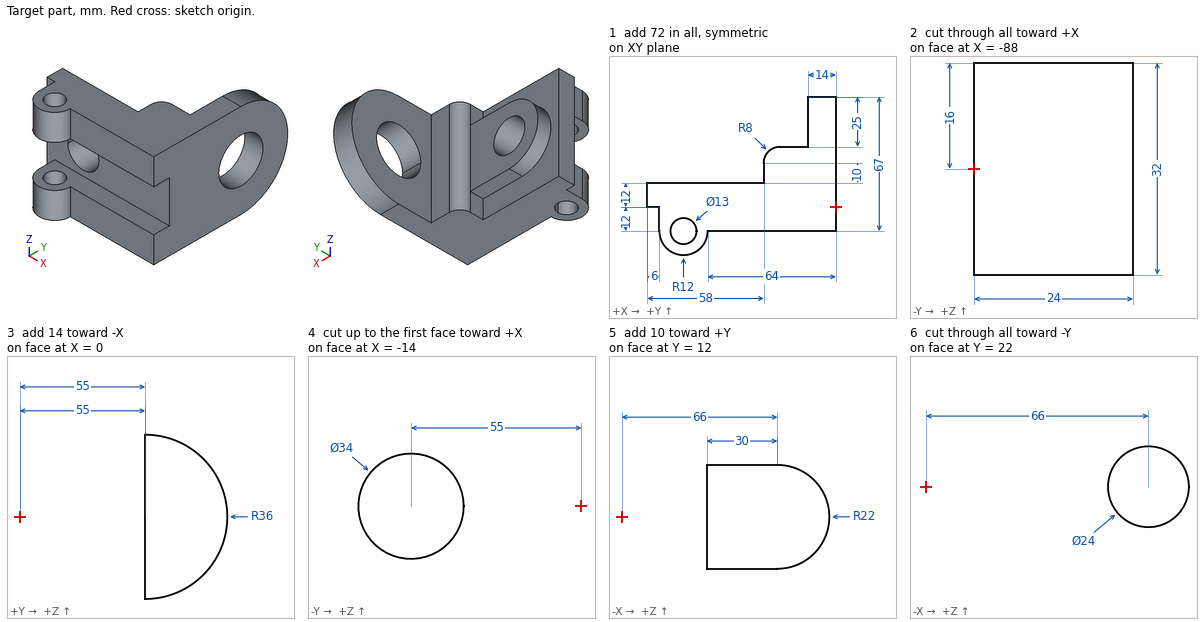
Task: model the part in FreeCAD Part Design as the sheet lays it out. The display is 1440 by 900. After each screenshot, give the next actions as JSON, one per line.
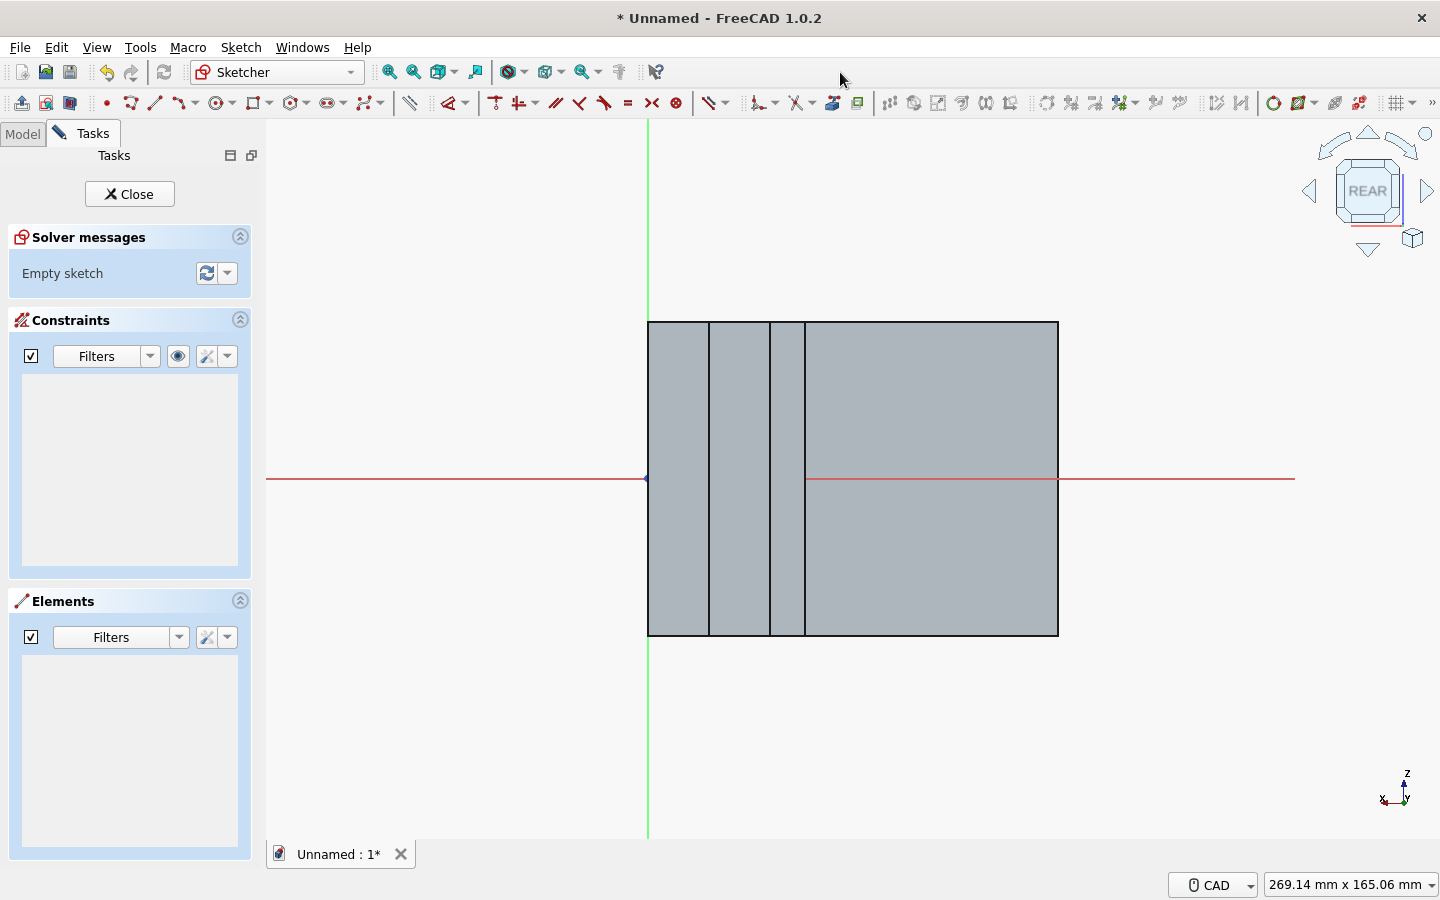
{"action": "scroll", "coordinate": [907, 479], "scroll_direction": "up", "scroll_amount": 3}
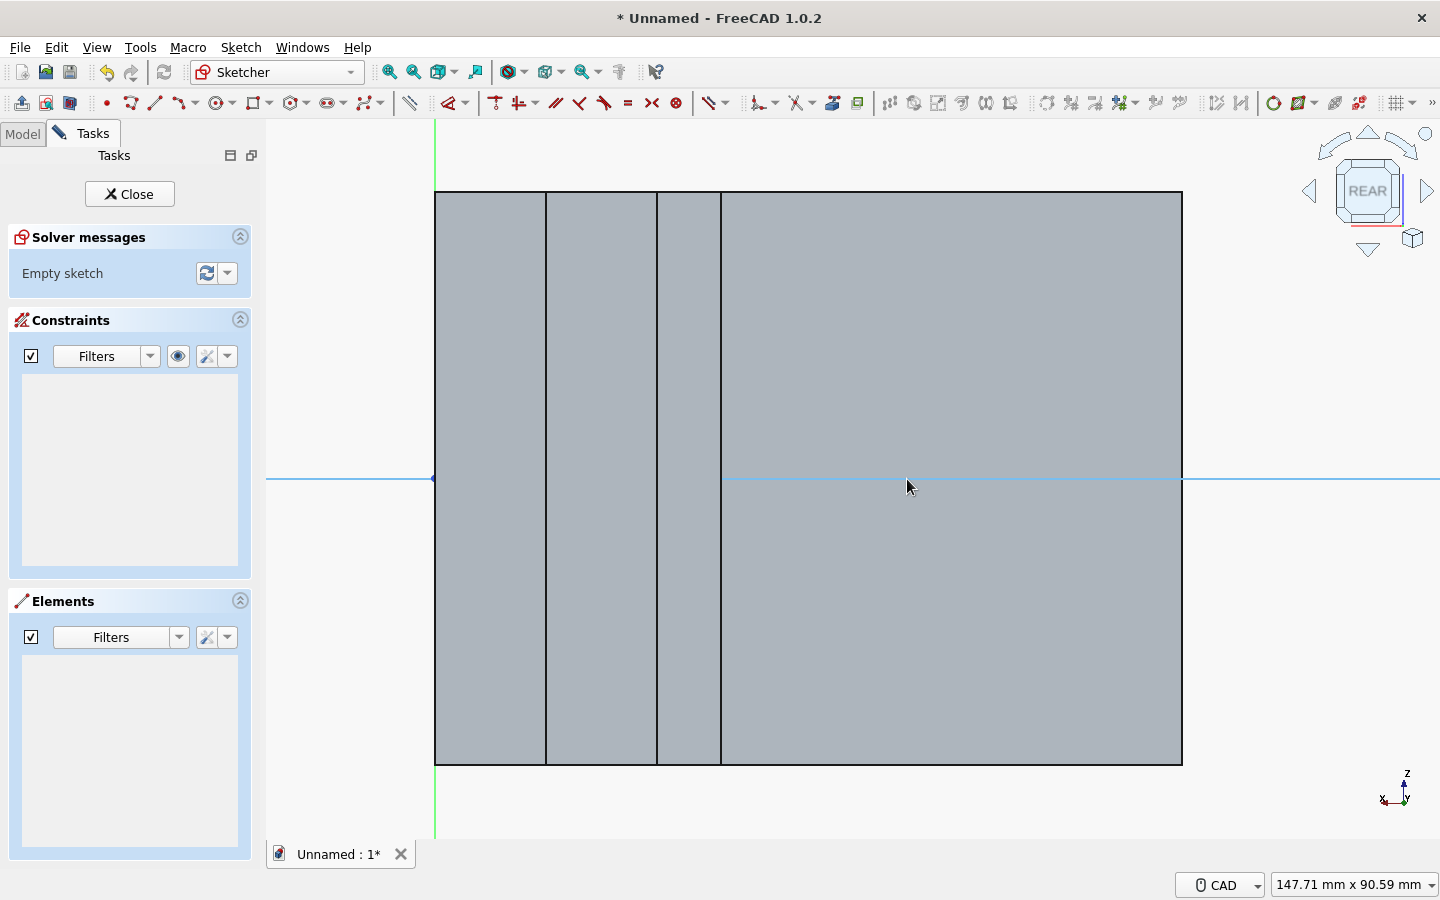
{"action": "left_click", "coordinate": [132, 104]}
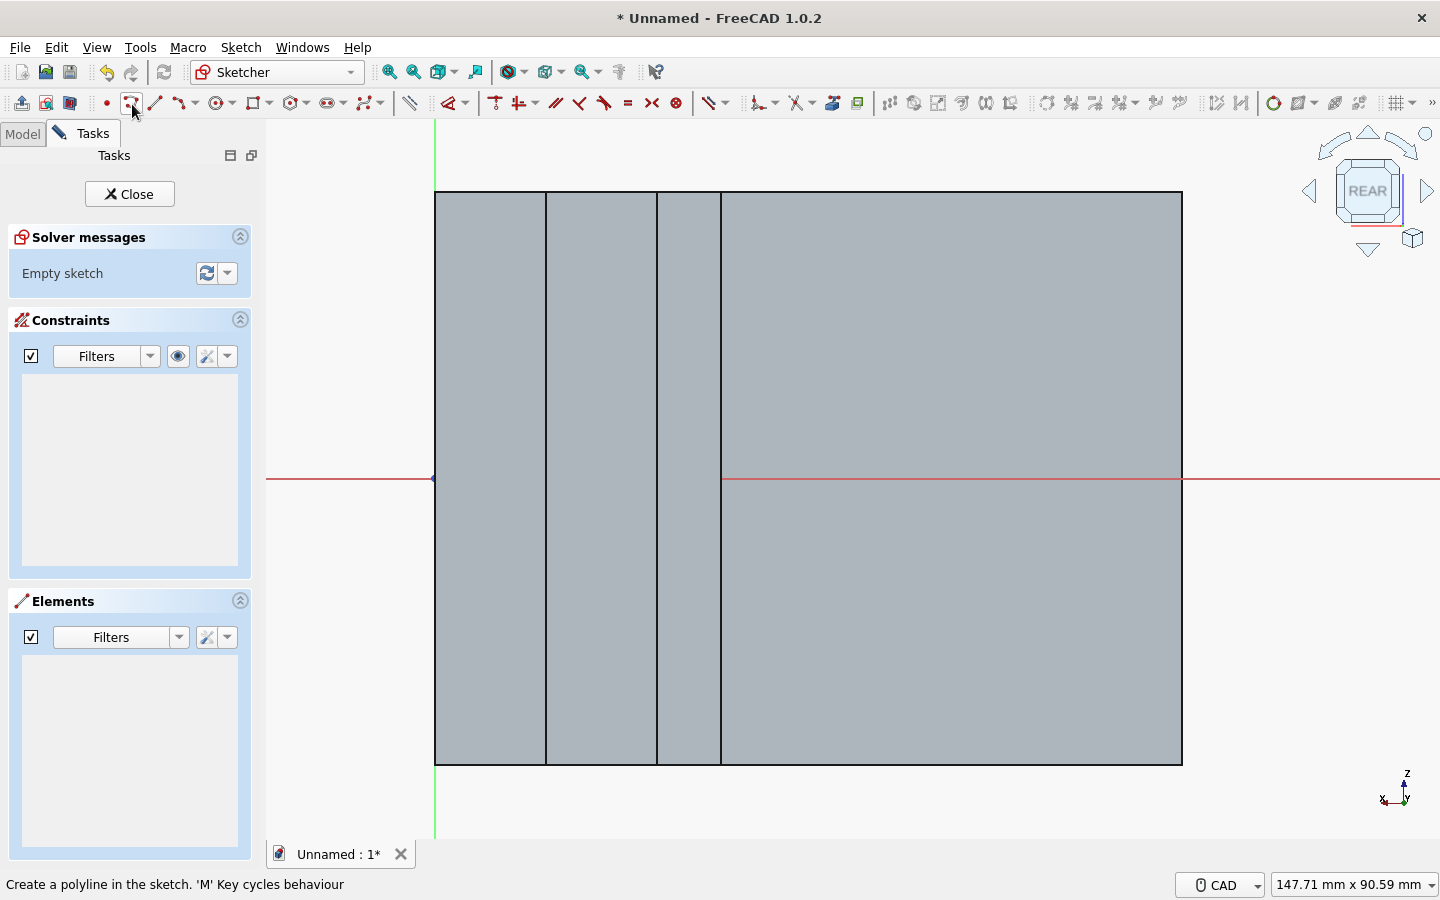
{"action": "left_click", "coordinate": [959, 304]}
{"action": "left_click", "coordinate": [721, 304]}
{"action": "left_click", "coordinate": [721, 653]}
{"action": "left_click", "coordinate": [959, 653]}
{"action": "right_click", "coordinate": [959, 653]}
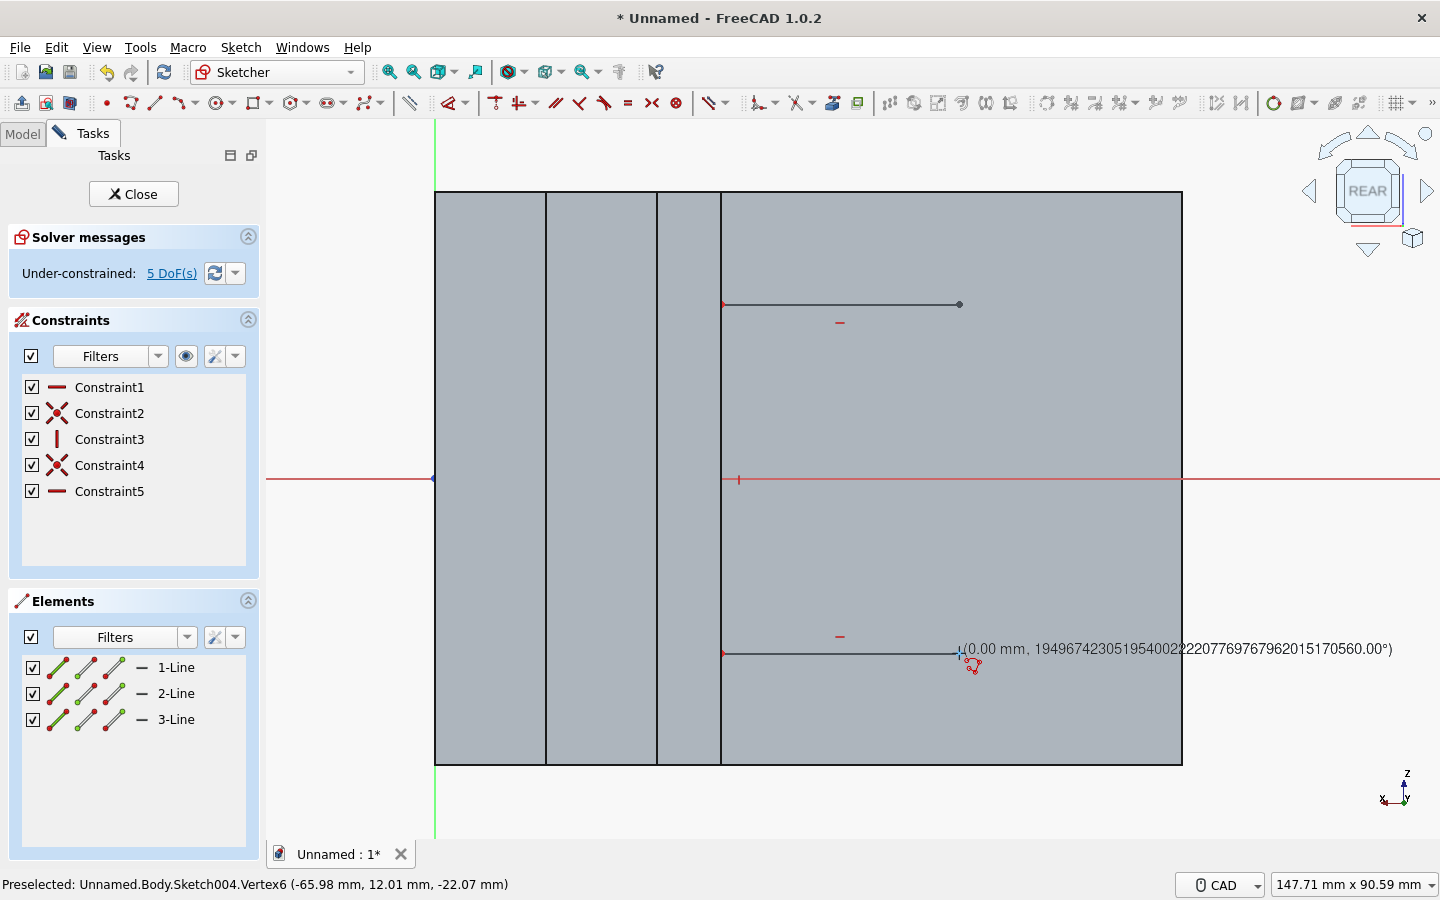
{"action": "left_click", "coordinate": [180, 104]}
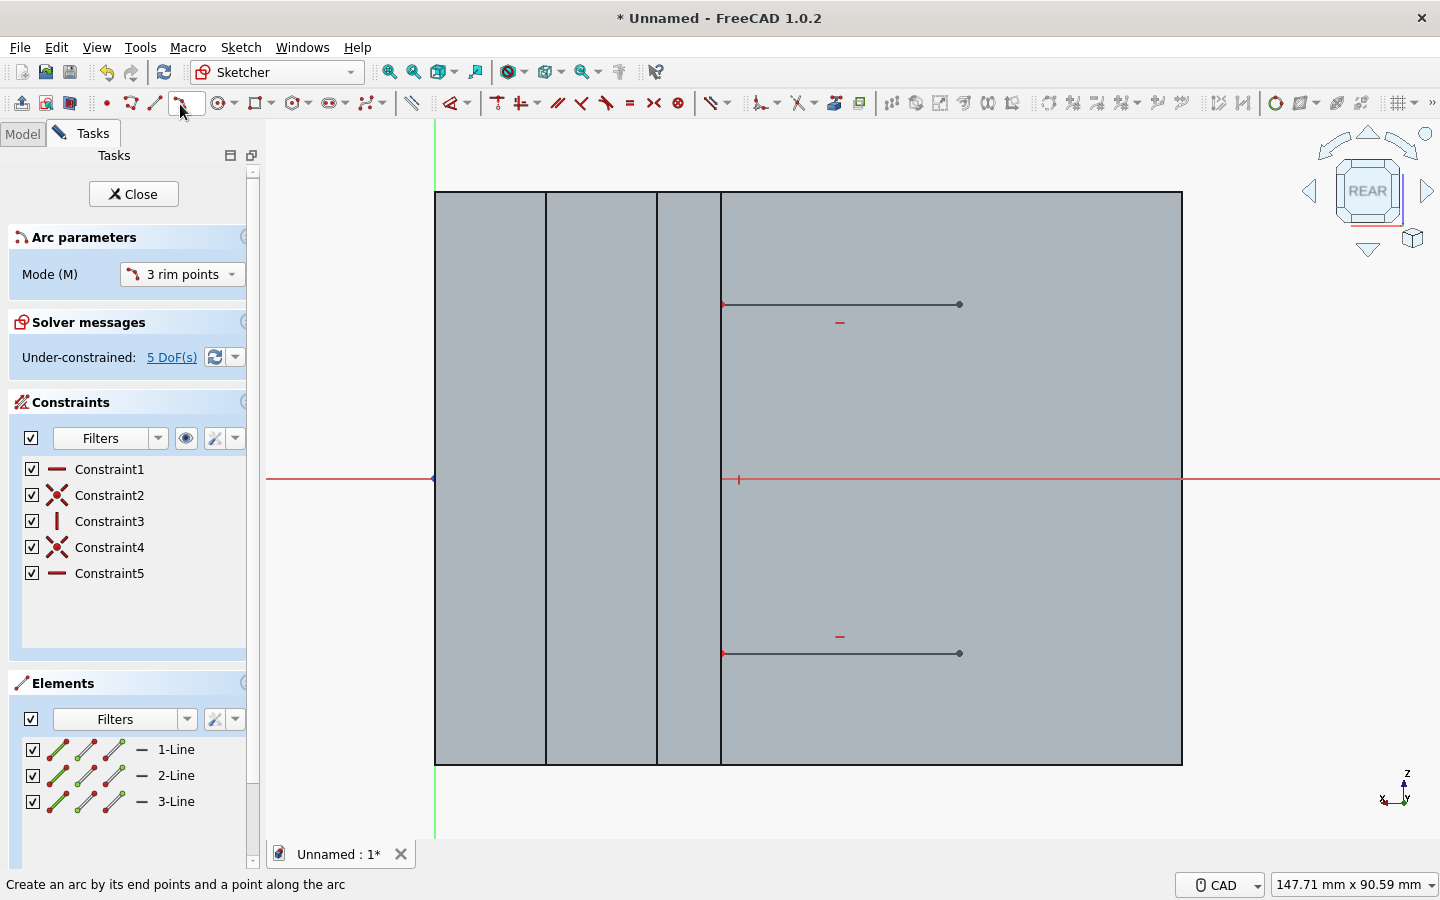
{"action": "left_click", "coordinate": [959, 654]}
{"action": "left_click", "coordinate": [959, 305]}
{"action": "left_click", "coordinate": [1125, 533]}
{"action": "key", "text": "Escape"}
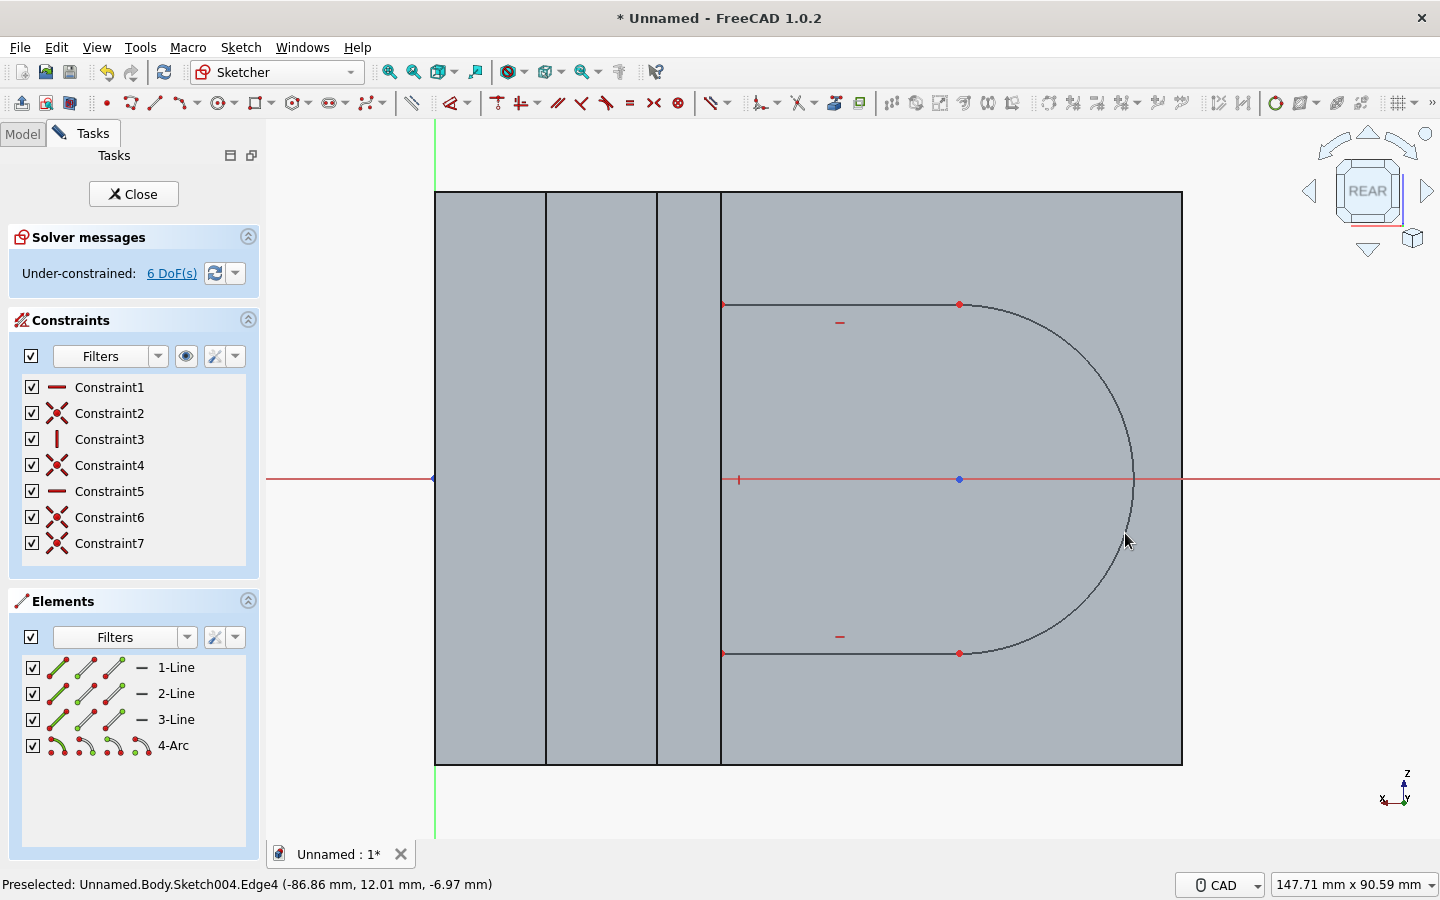
{"action": "left_click", "coordinate": [888, 305]}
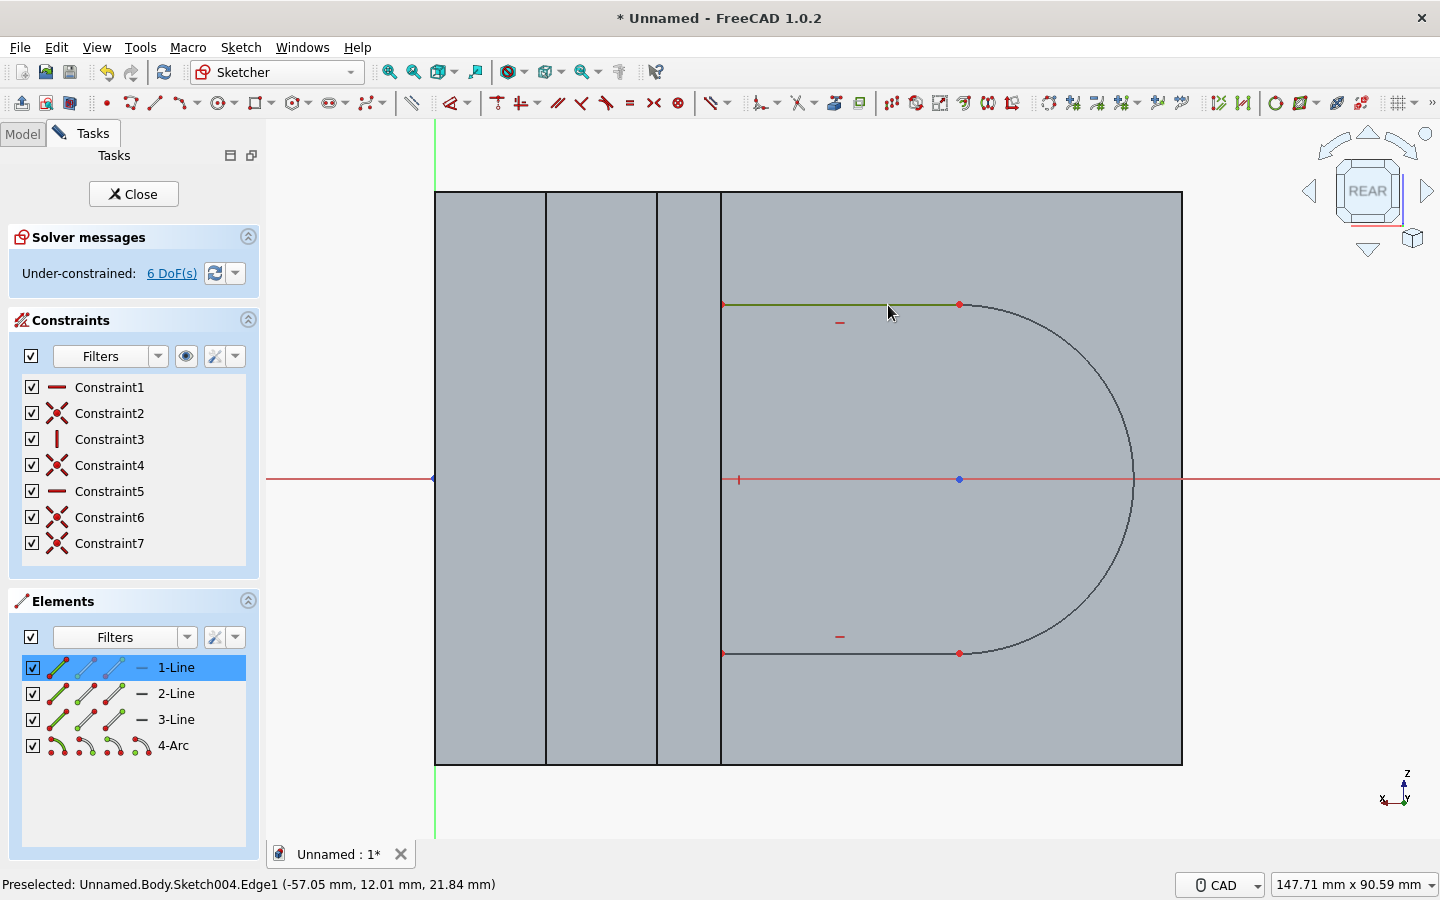
{"action": "left_click", "coordinate": [1100, 582]}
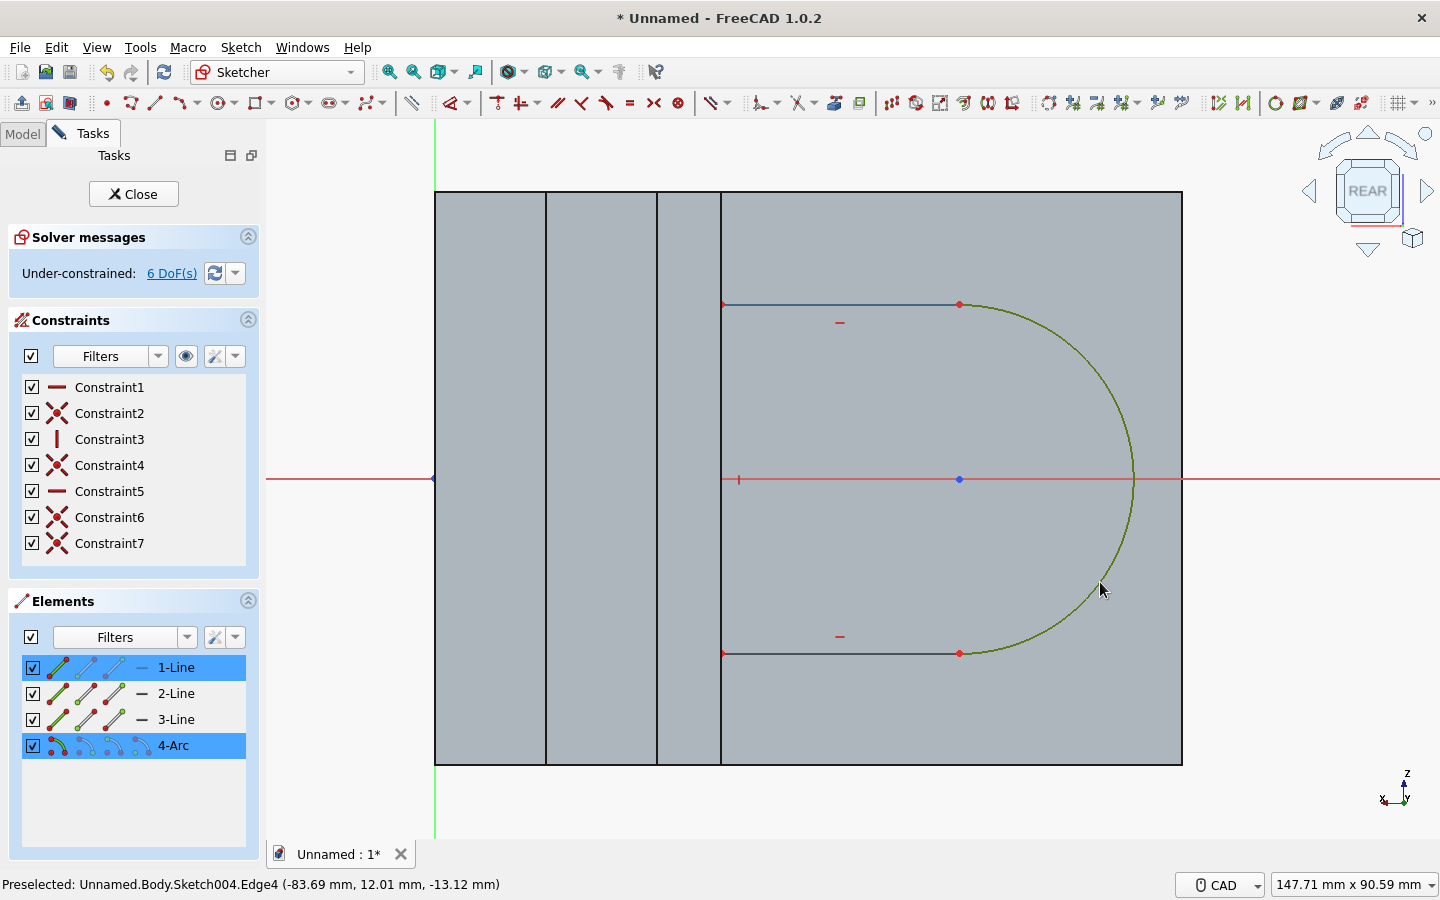
{"action": "left_click", "coordinate": [606, 104]}